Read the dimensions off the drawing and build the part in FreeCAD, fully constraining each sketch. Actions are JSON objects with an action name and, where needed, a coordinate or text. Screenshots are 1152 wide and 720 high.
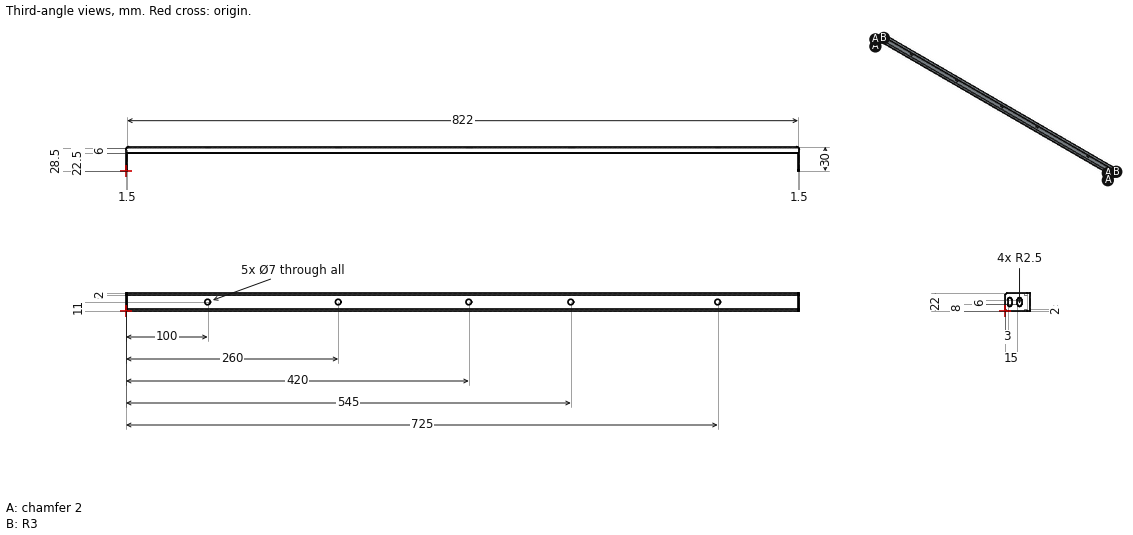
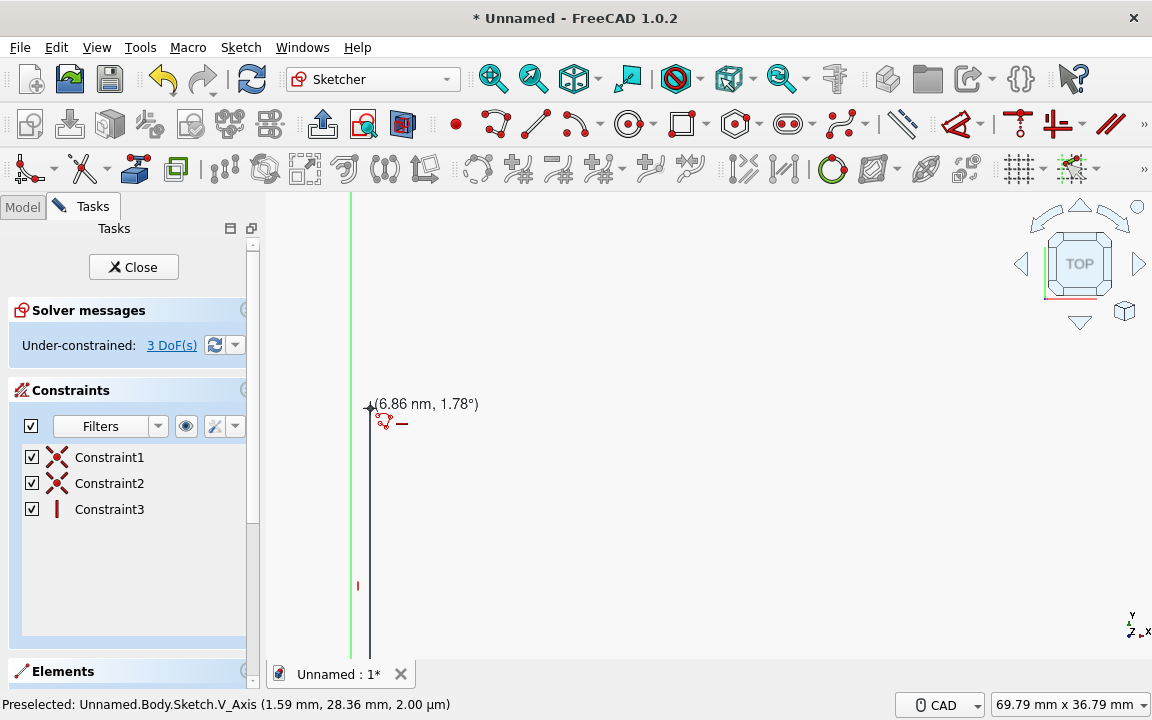
{"action": "scroll", "coordinate": [381, 417], "scroll_direction": "down", "scroll_amount": 15}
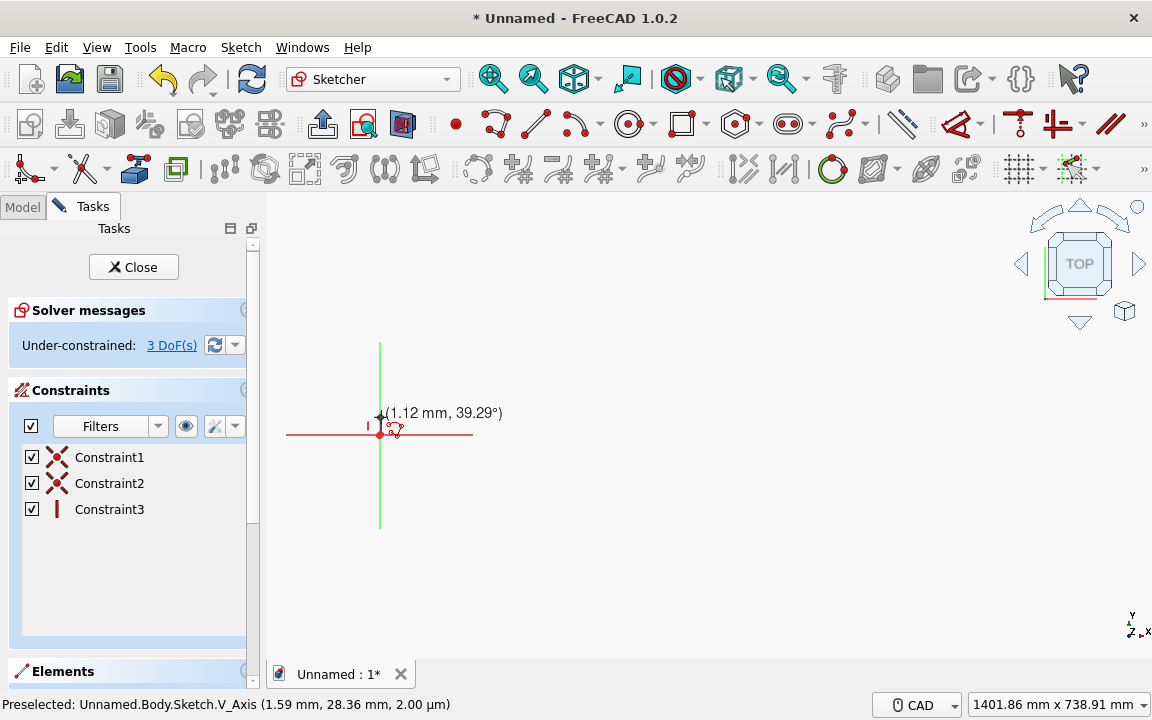
{"action": "left_click", "coordinate": [900, 417]}
{"action": "left_click", "coordinate": [900, 435]}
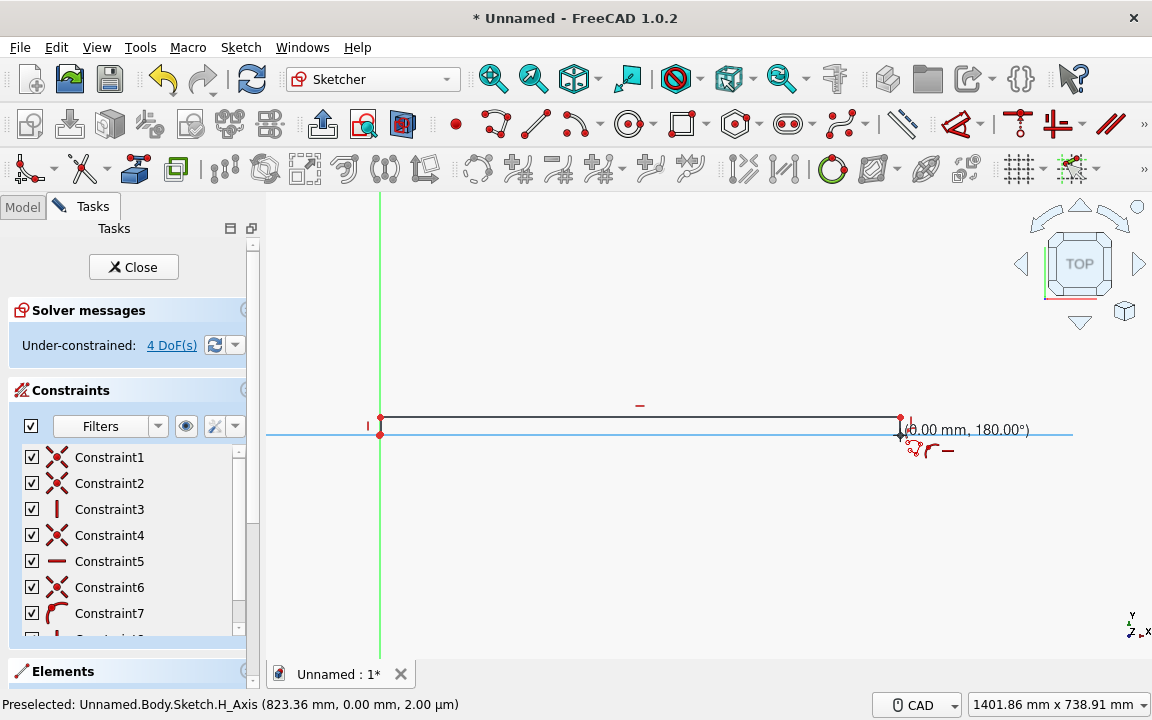
{"action": "scroll", "coordinate": [901, 435], "scroll_direction": "up", "scroll_amount": 15}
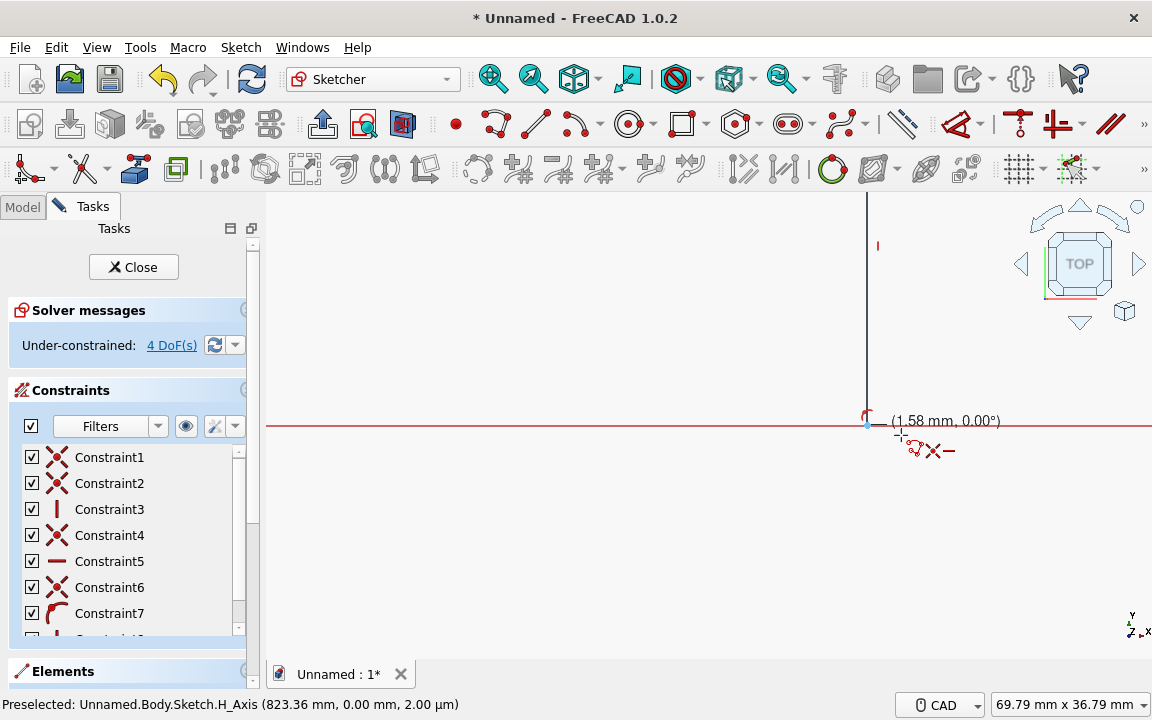
{"action": "left_click", "coordinate": [888, 417]}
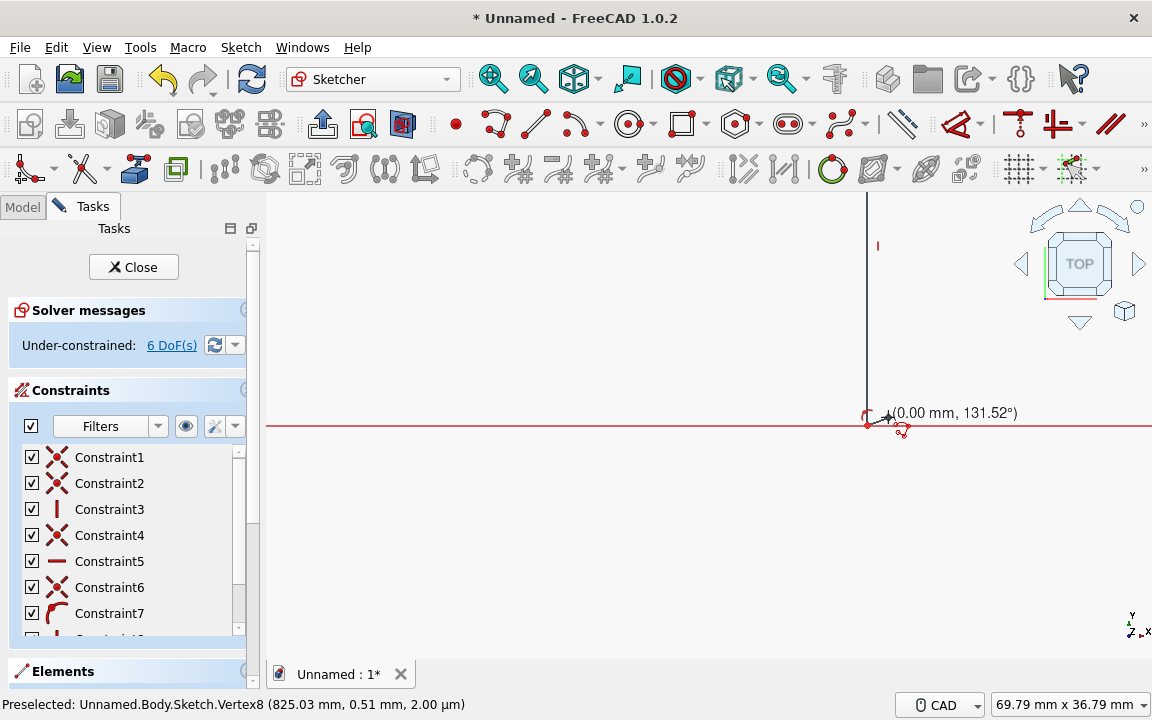
{"action": "scroll", "coordinate": [902, 435], "scroll_direction": "down", "scroll_amount": 15}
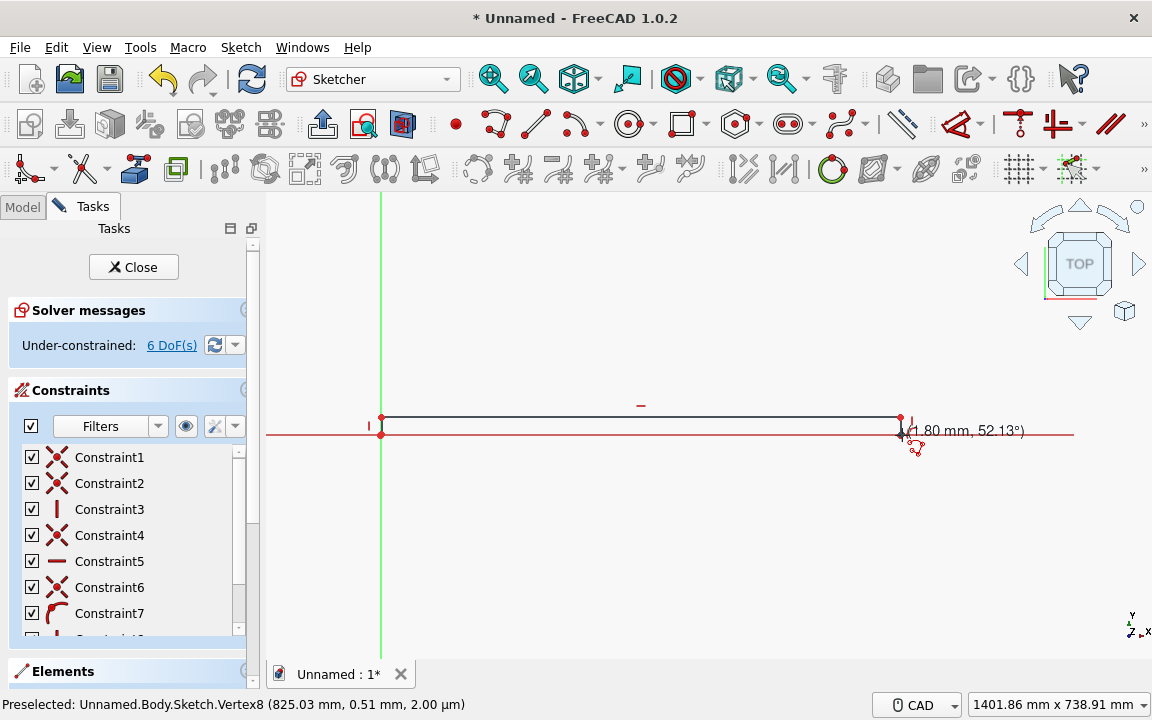
{"action": "scroll", "coordinate": [902, 416], "scroll_direction": "up", "scroll_amount": 13}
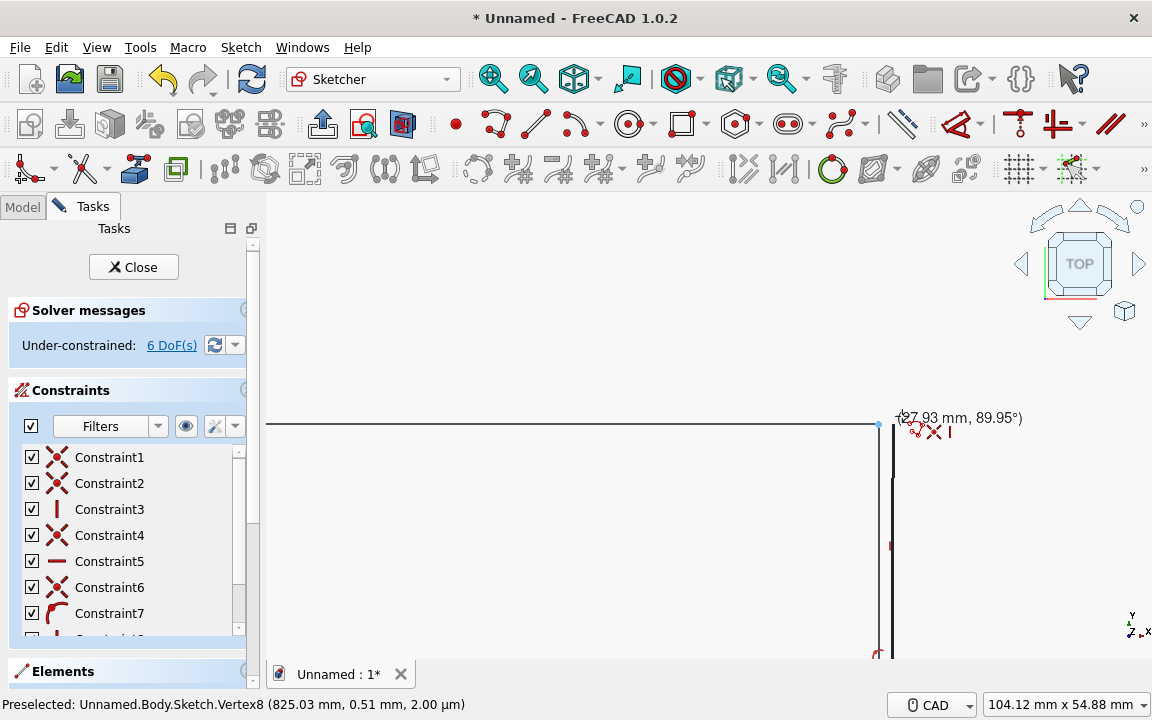
{"action": "left_click", "coordinate": [893, 411]}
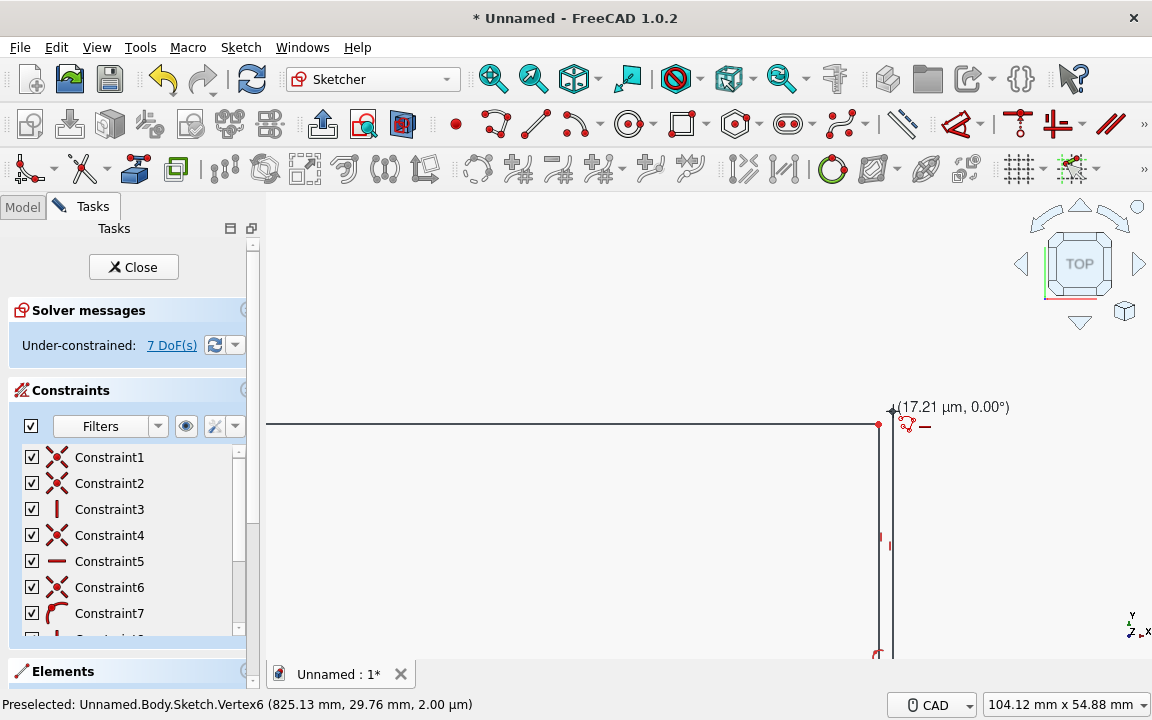
{"action": "scroll", "coordinate": [902, 416], "scroll_direction": "down", "scroll_amount": 13}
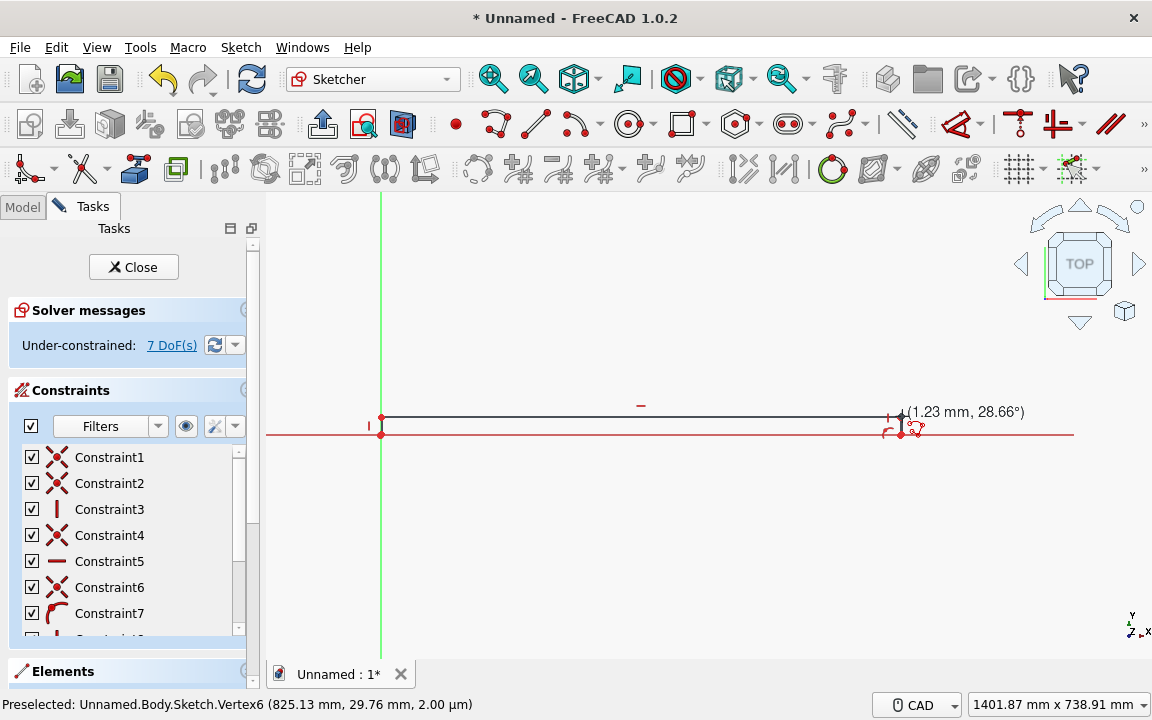
{"action": "scroll", "coordinate": [381, 416], "scroll_direction": "up", "scroll_amount": 13}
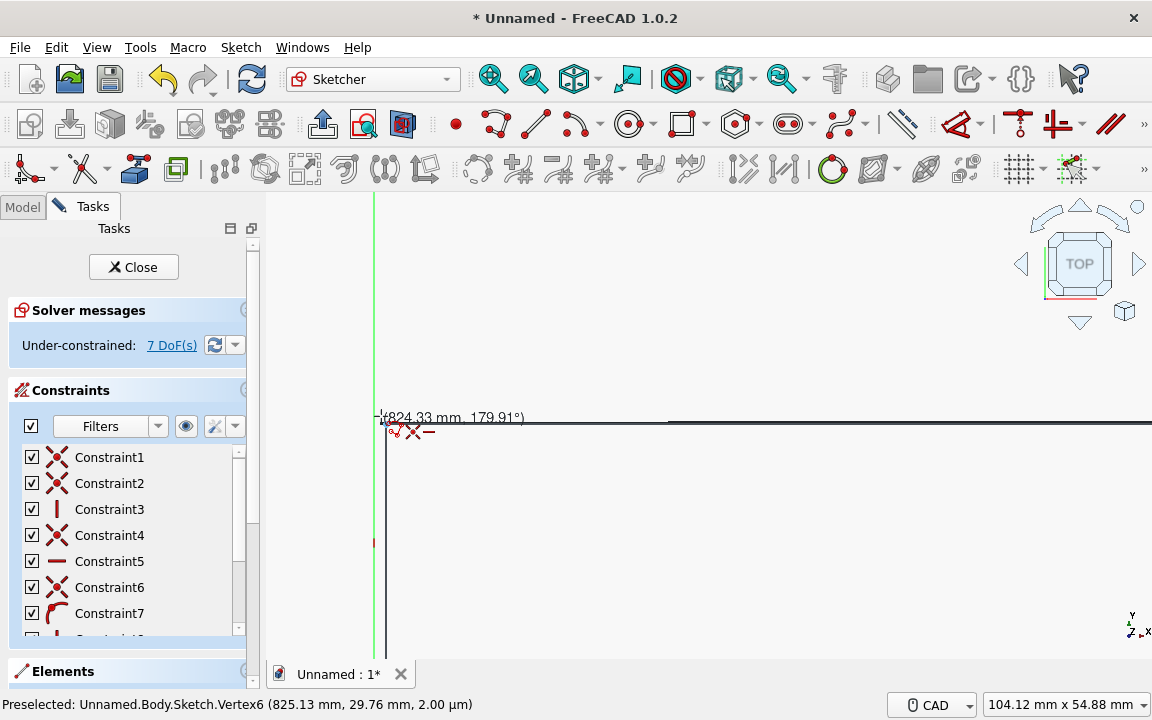
{"action": "left_click", "coordinate": [383, 411]}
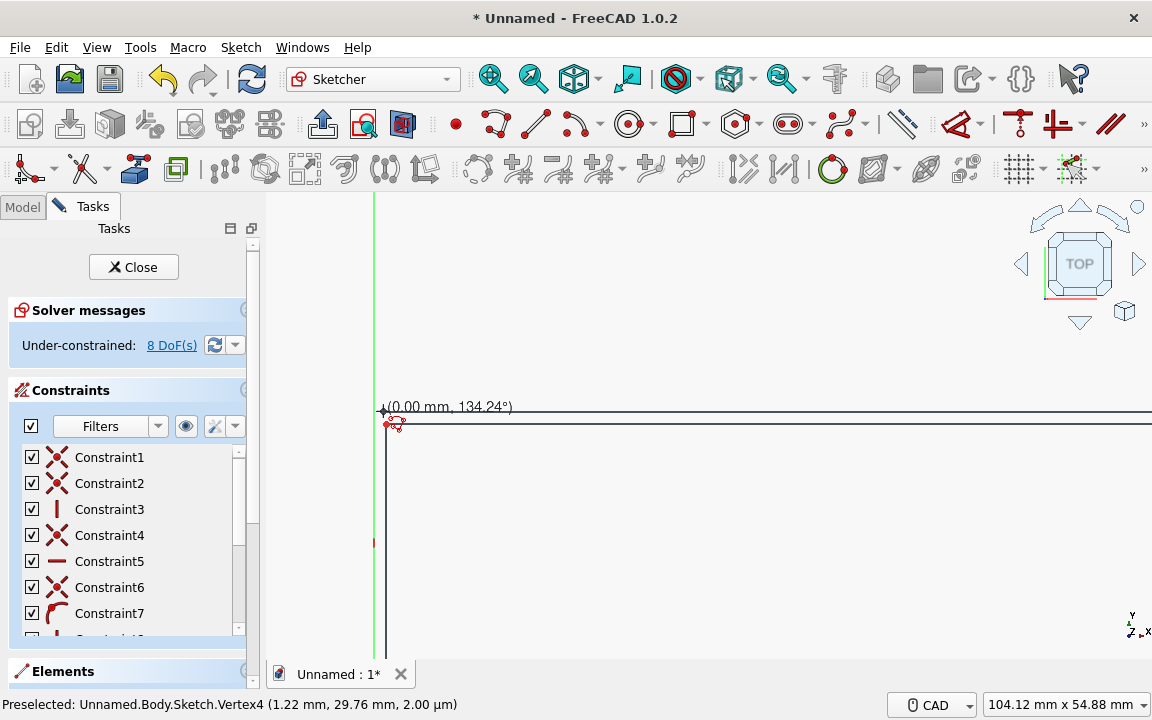
{"action": "scroll", "coordinate": [380, 416], "scroll_direction": "down", "scroll_amount": 13}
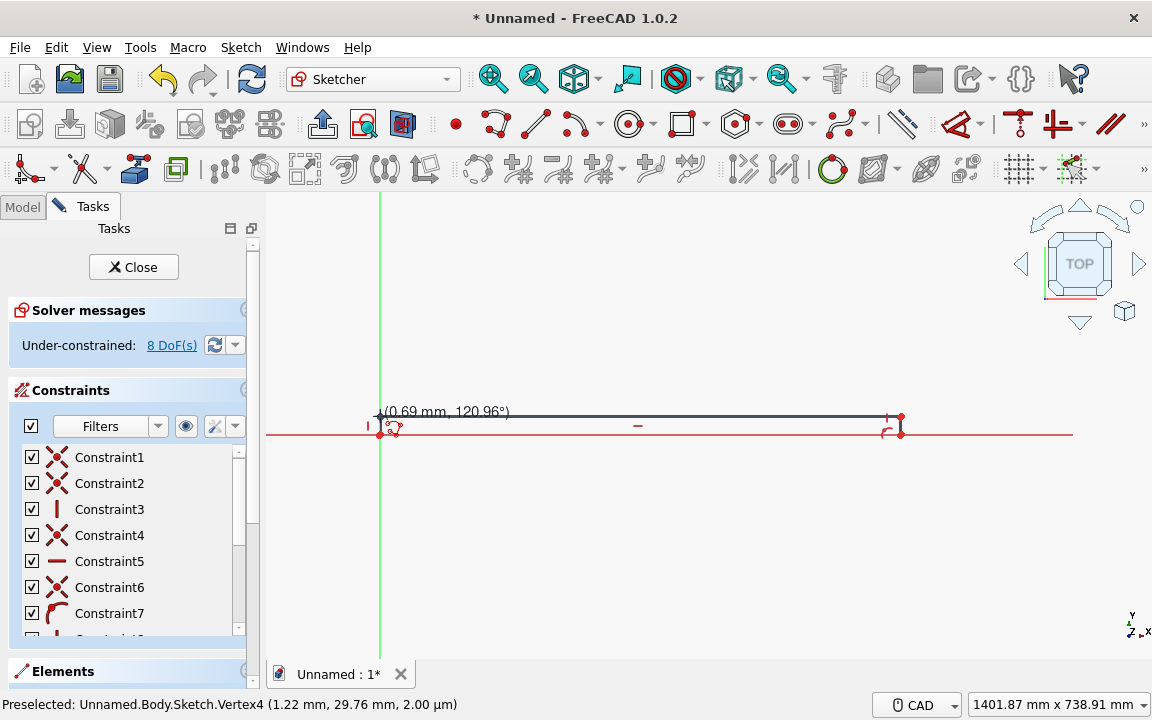
{"action": "scroll", "coordinate": [380, 435], "scroll_direction": "up", "scroll_amount": 18}